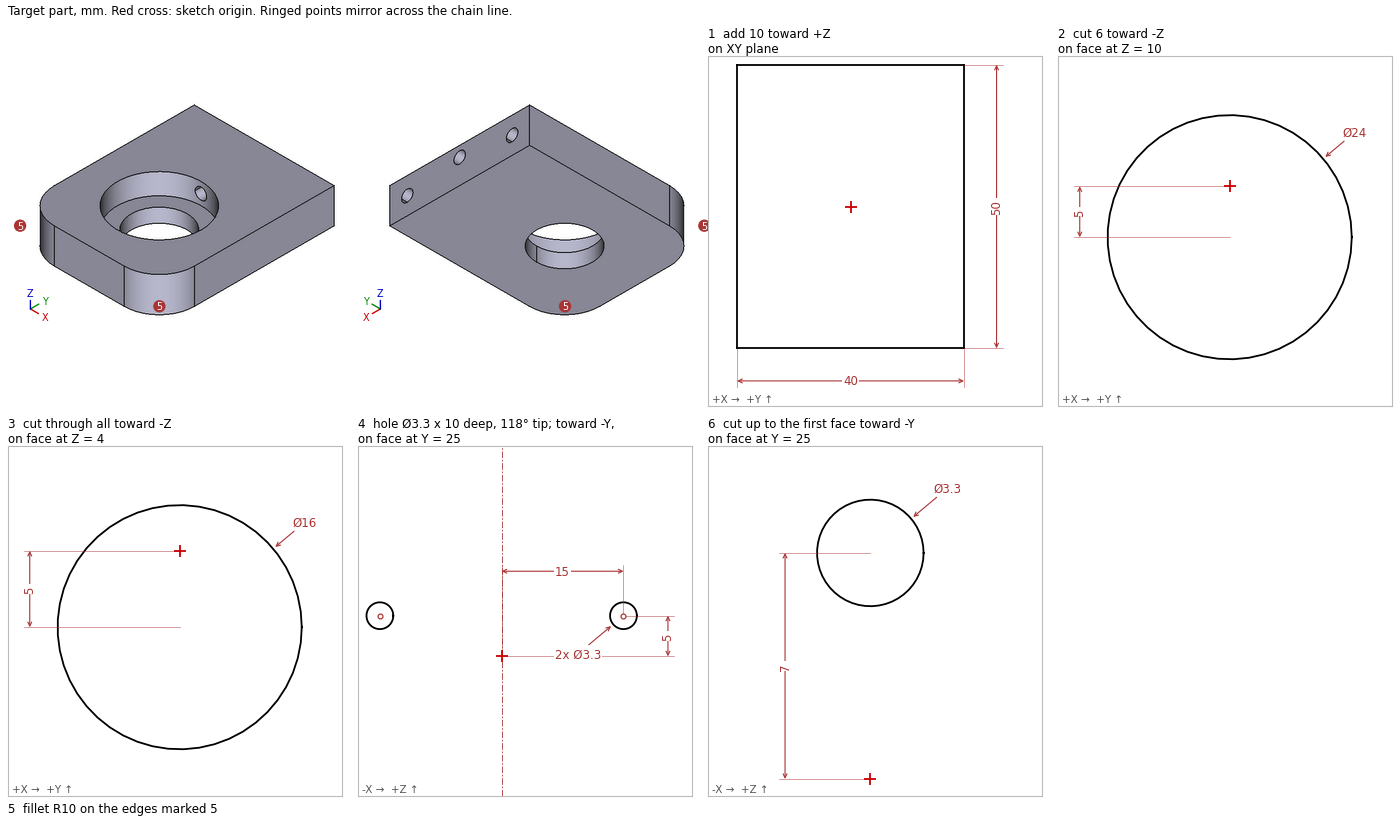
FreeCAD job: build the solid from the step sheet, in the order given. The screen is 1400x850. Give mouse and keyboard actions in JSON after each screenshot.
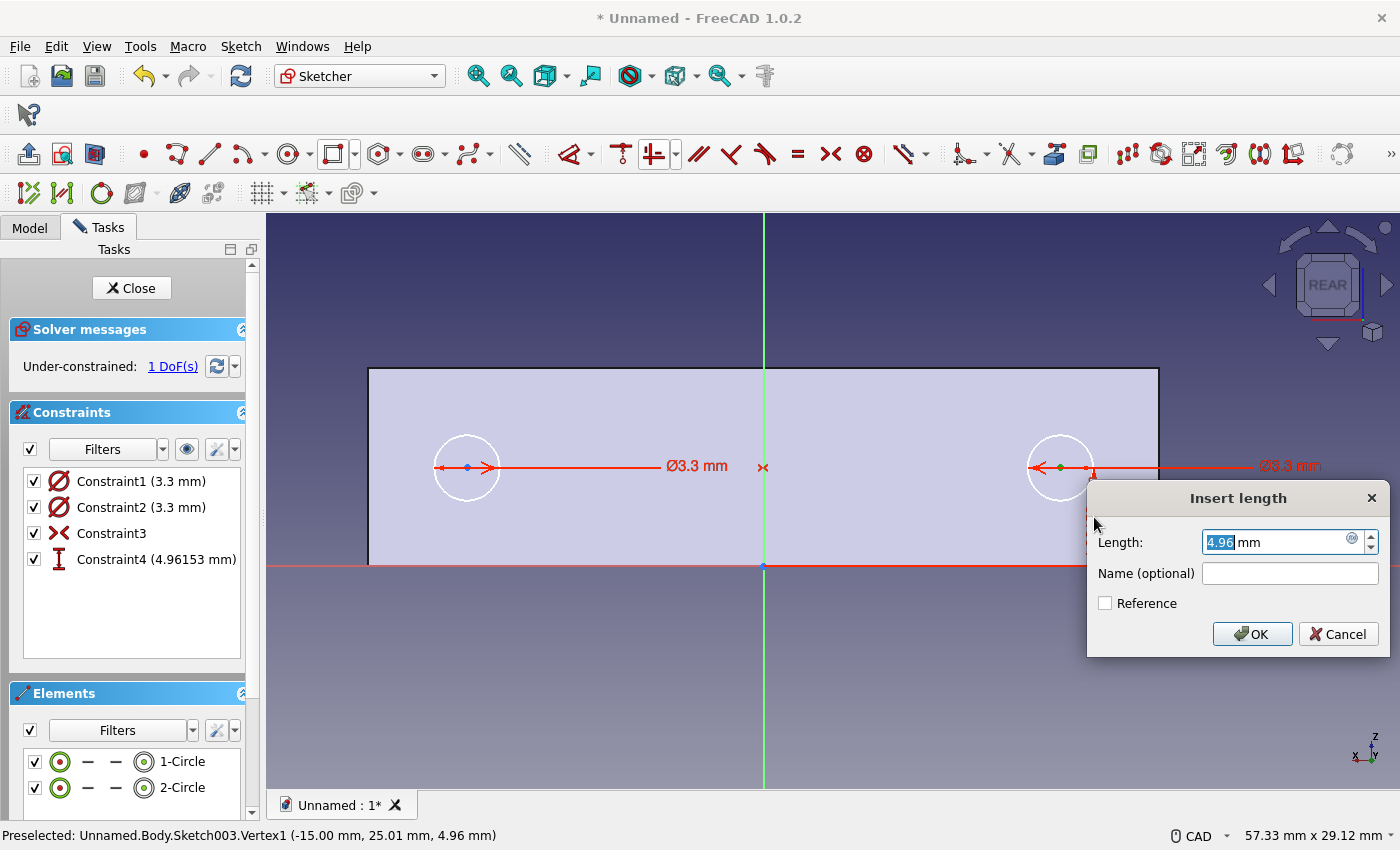
{"action": "type", "text": "5"}
{"action": "key", "text": "Return"}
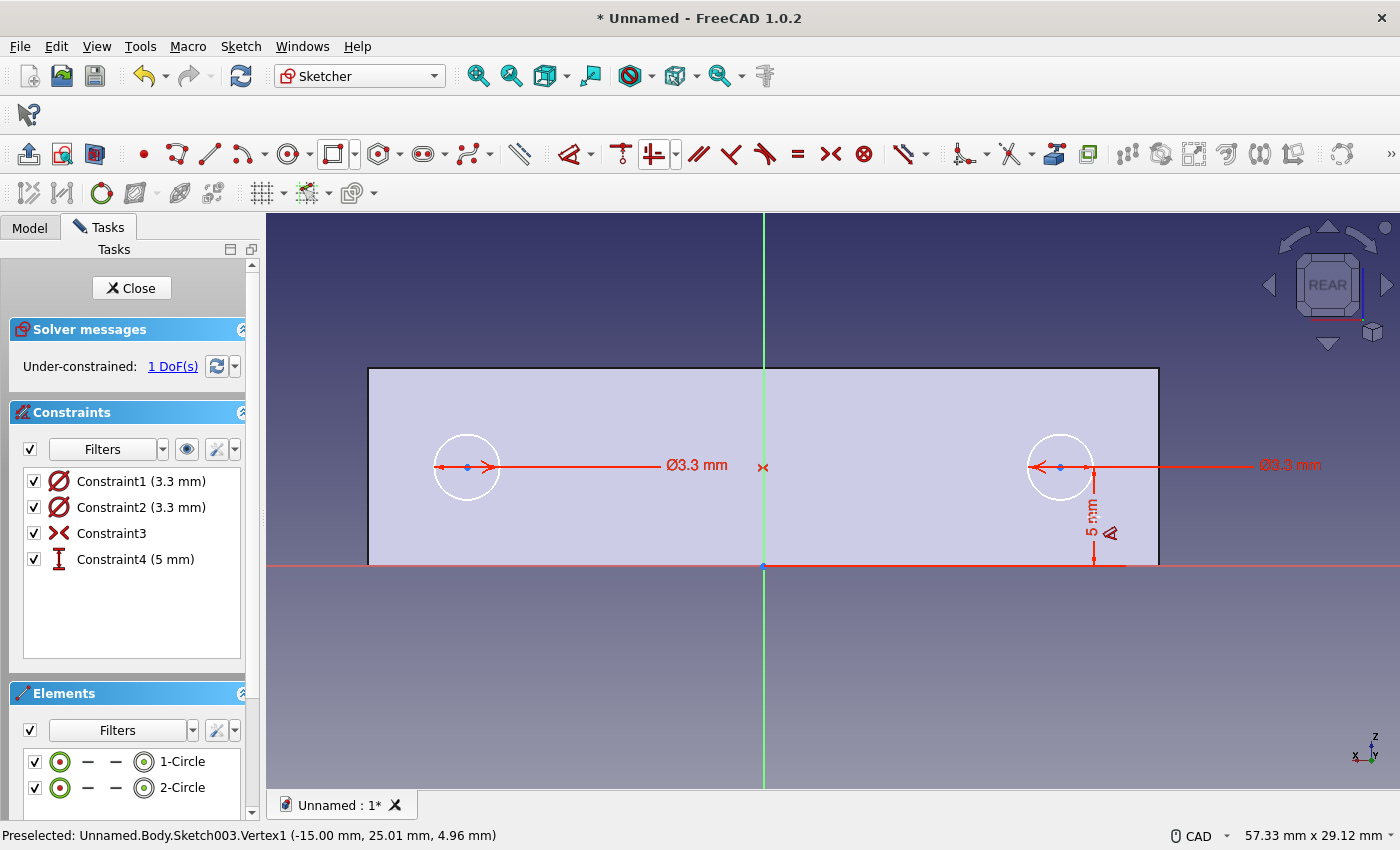
{"action": "left_click", "coordinate": [1060, 467]}
{"action": "left_click", "coordinate": [912, 600]}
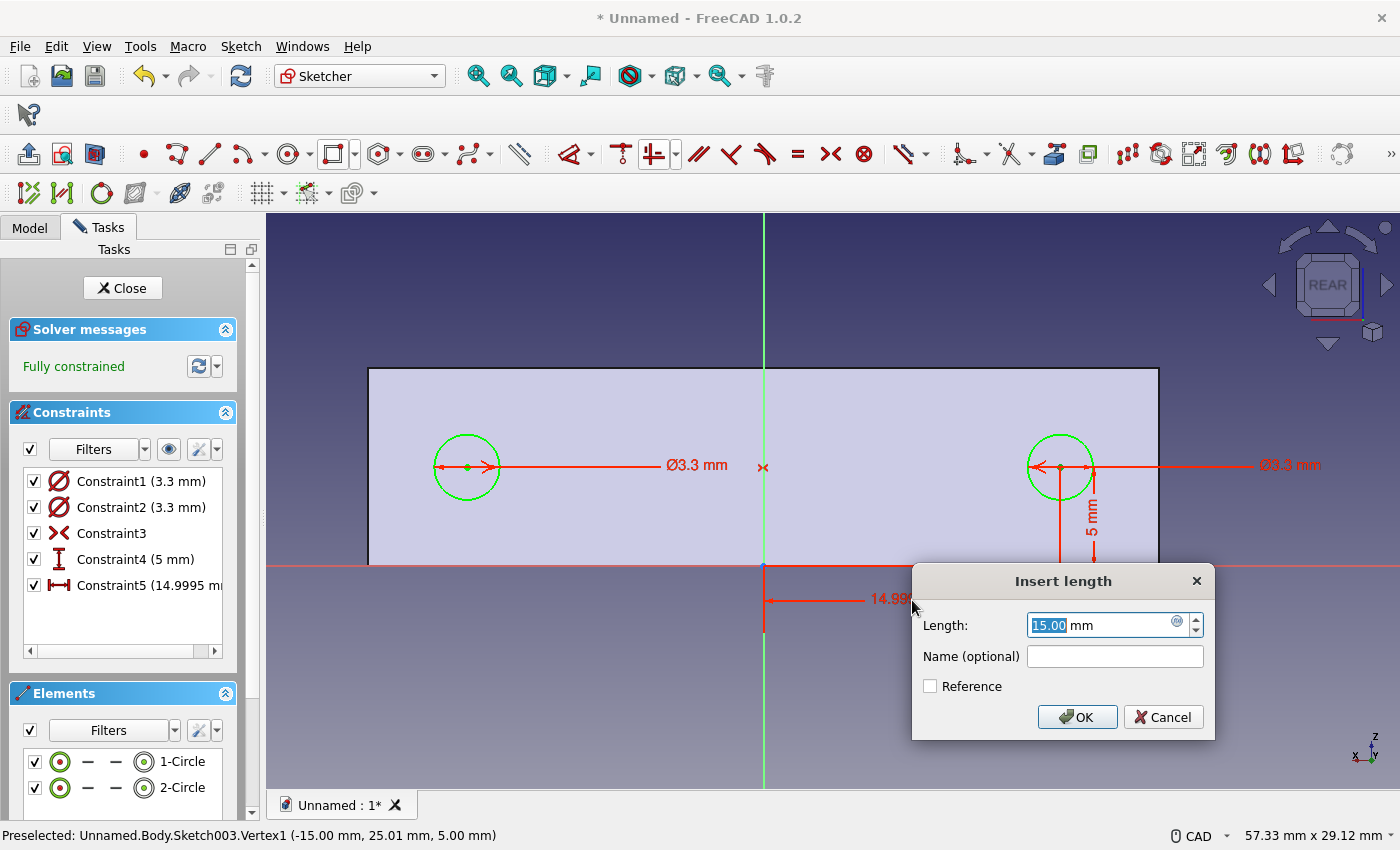
{"action": "type", "text": "15"}
{"action": "key", "text": "Return"}
{"action": "key", "text": "Escape"}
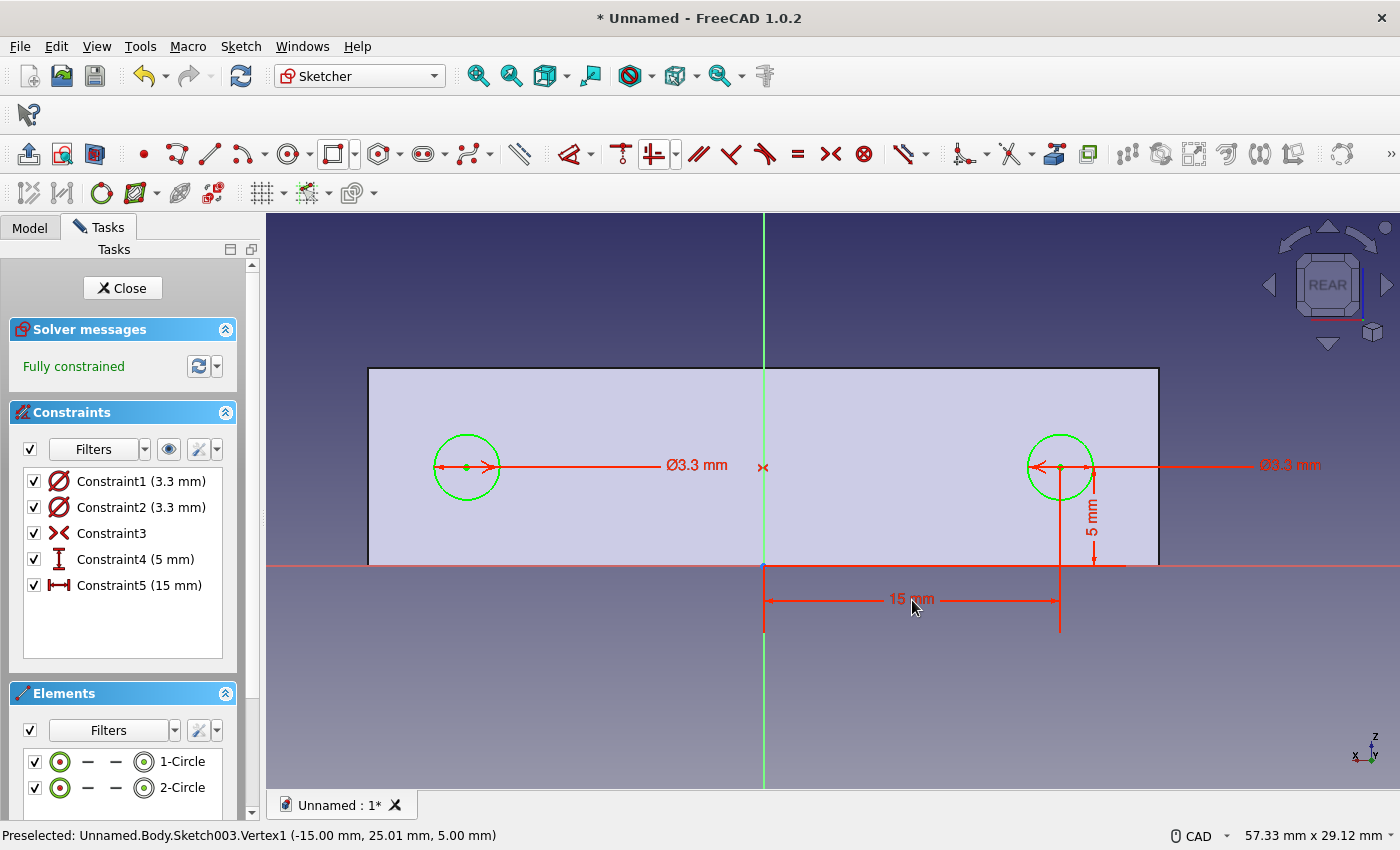
{"action": "left_click", "coordinate": [123, 288]}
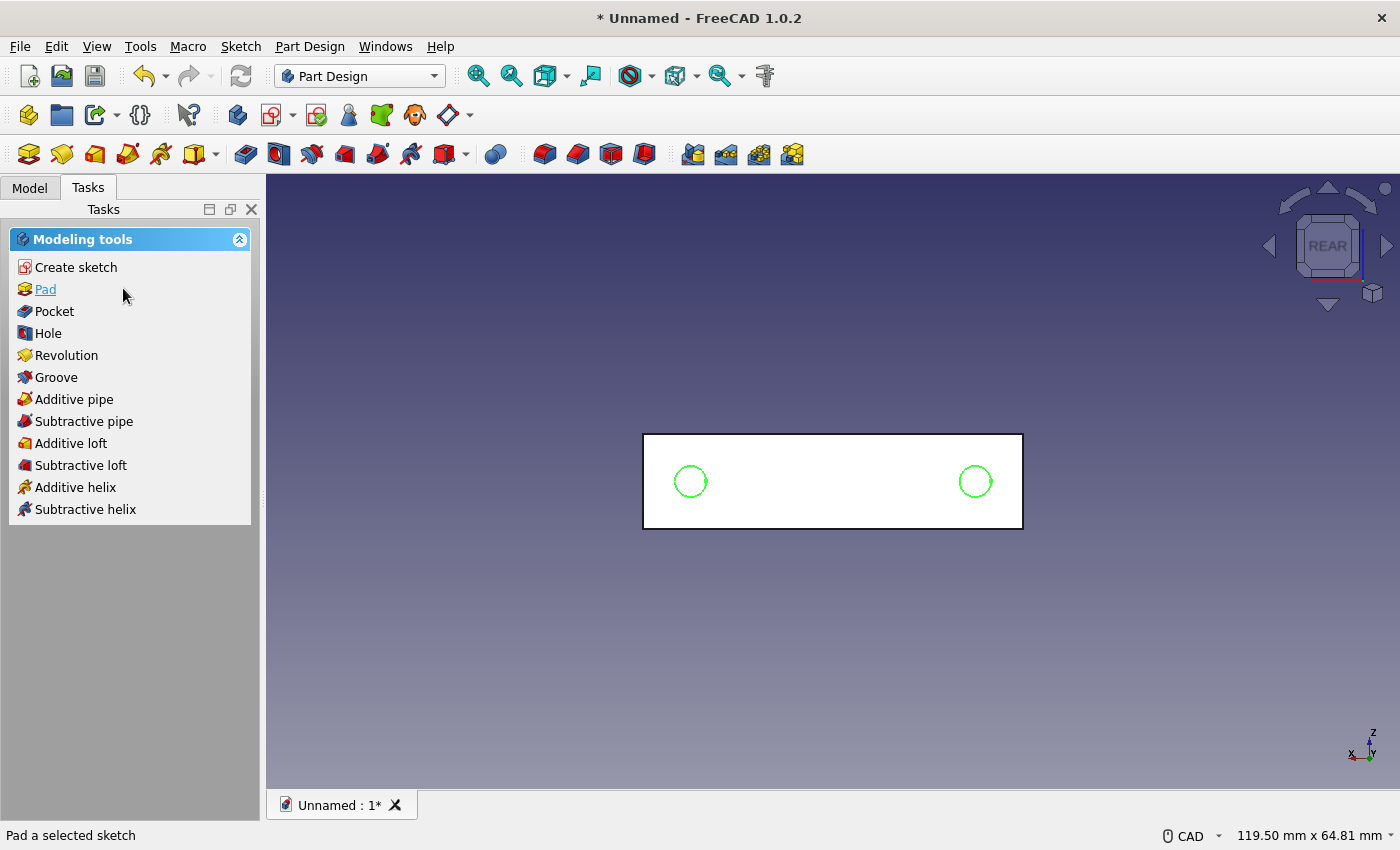
{"action": "left_click", "coordinate": [279, 154]}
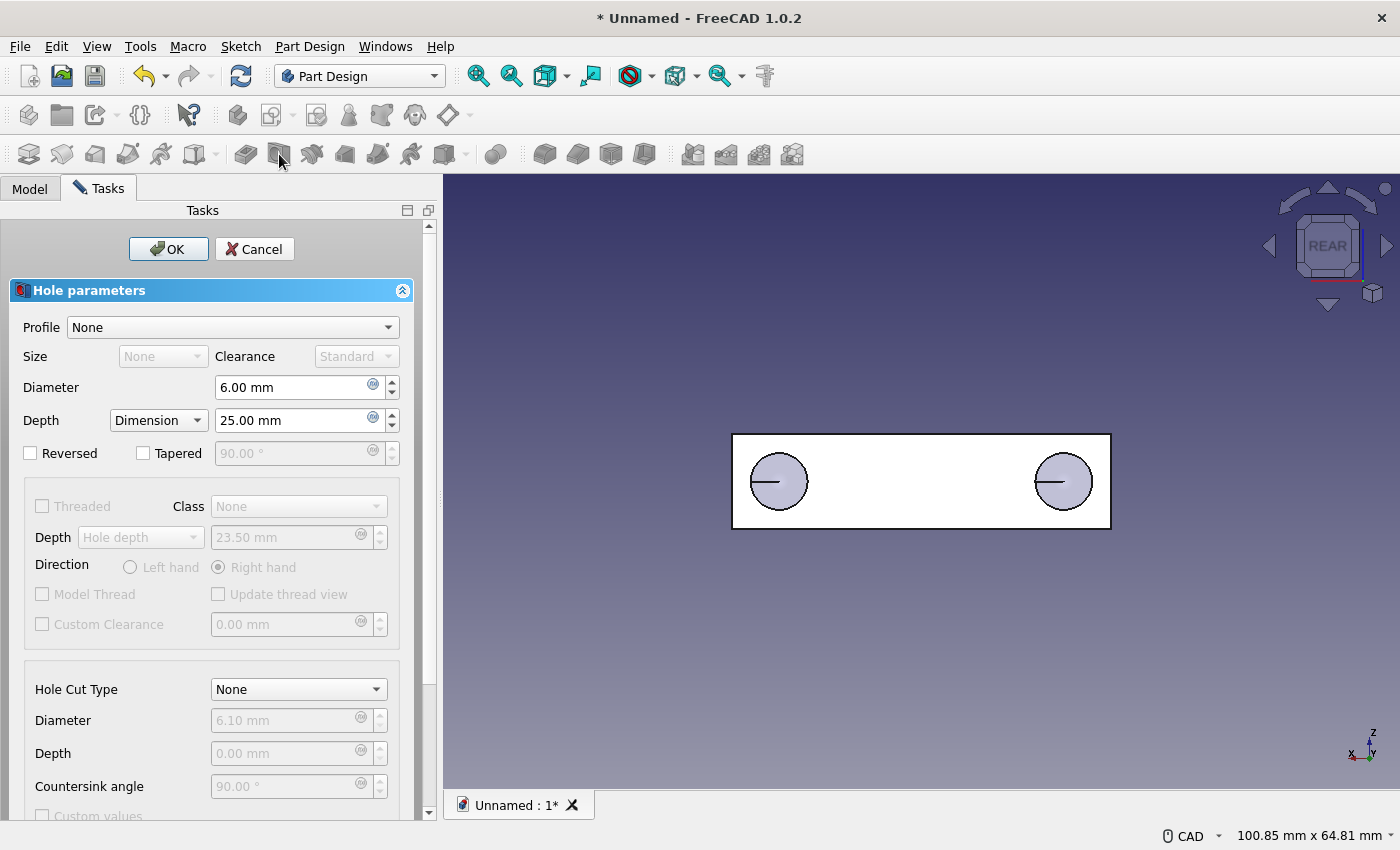
{"action": "triple_click", "coordinate": [300, 388]}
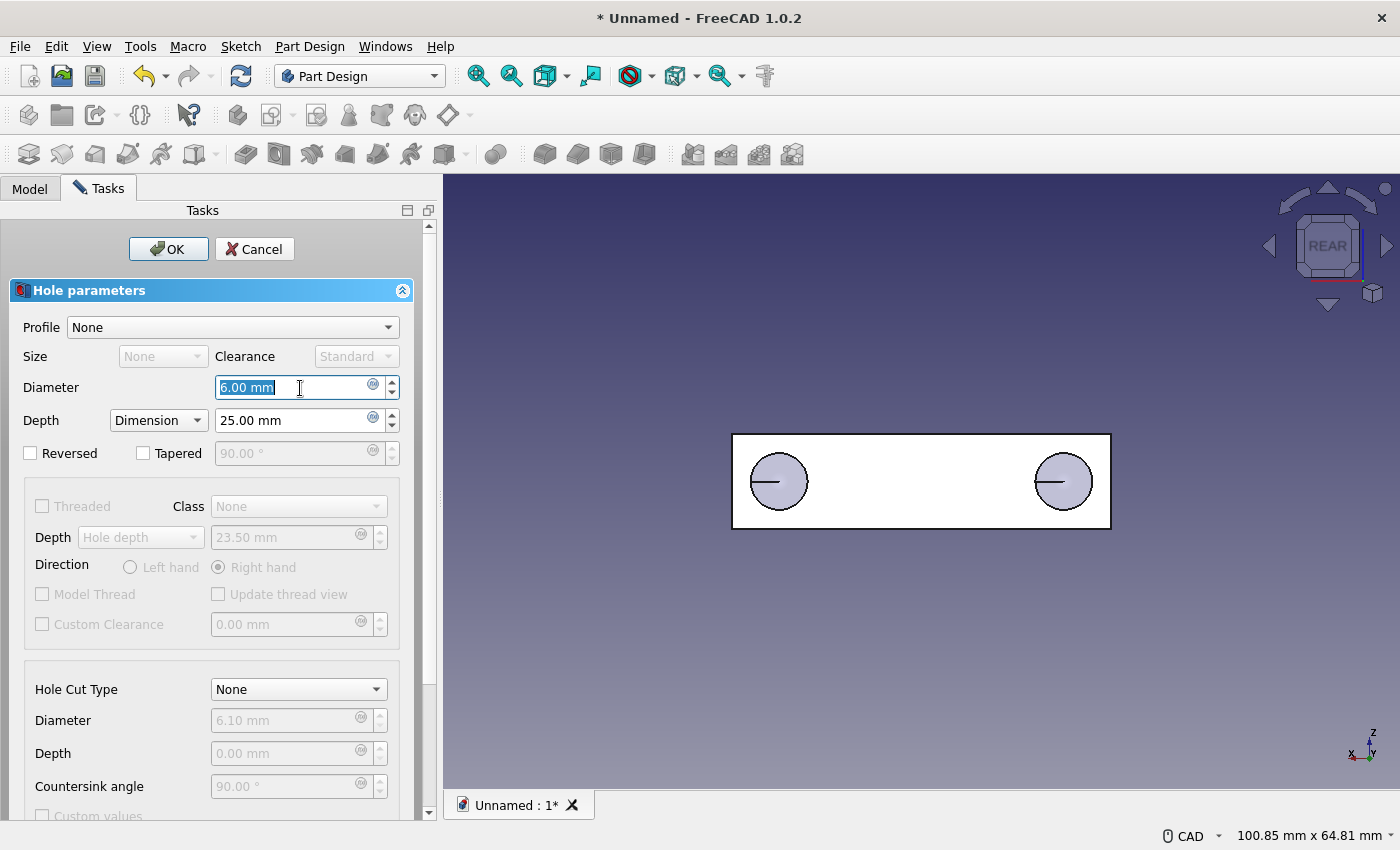
{"action": "type", "text": "3.3"}
{"action": "key", "text": "Tab"}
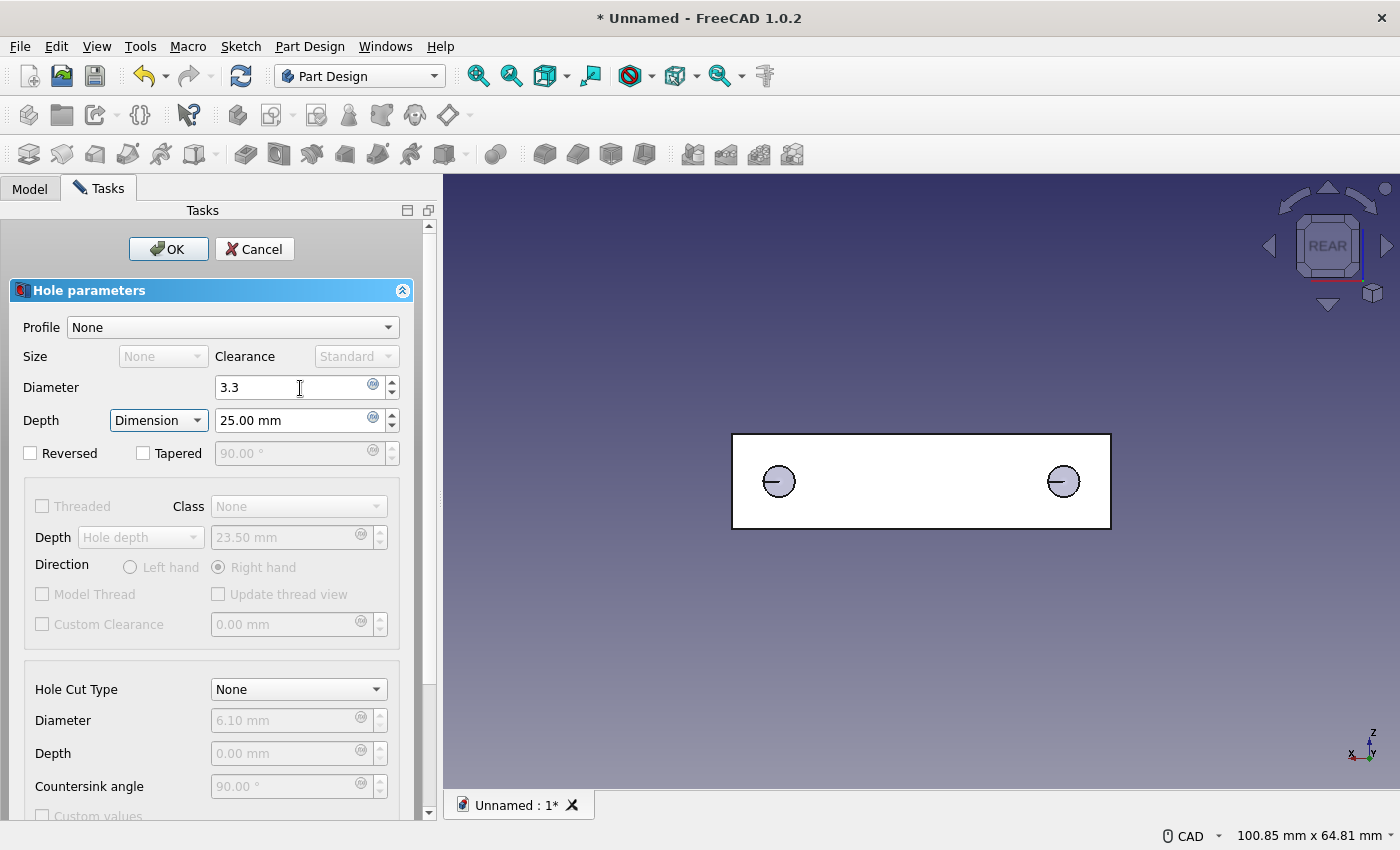
{"action": "triple_click", "coordinate": [300, 420]}